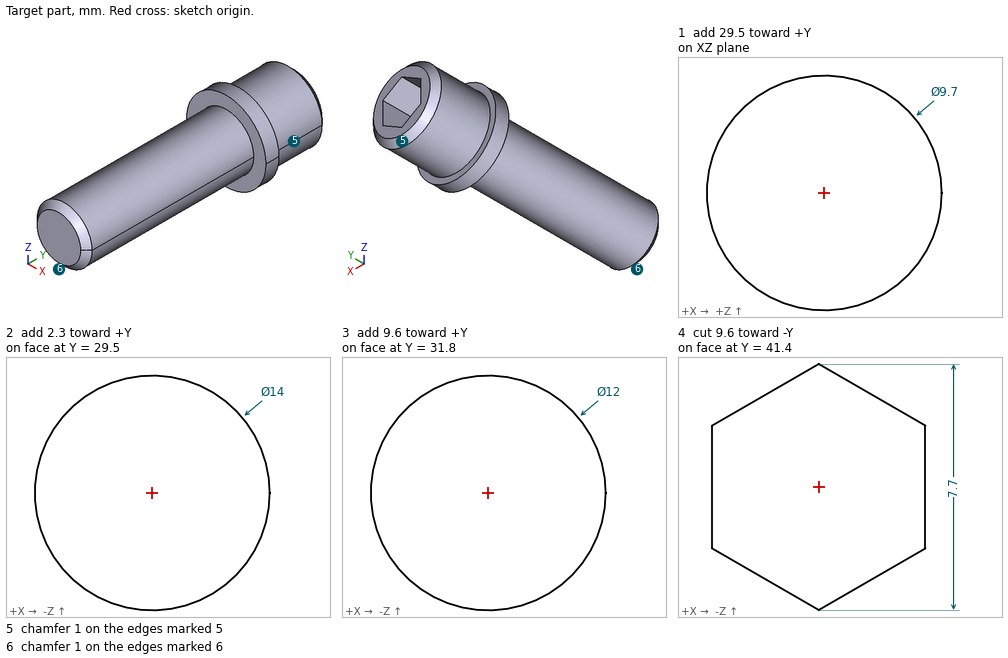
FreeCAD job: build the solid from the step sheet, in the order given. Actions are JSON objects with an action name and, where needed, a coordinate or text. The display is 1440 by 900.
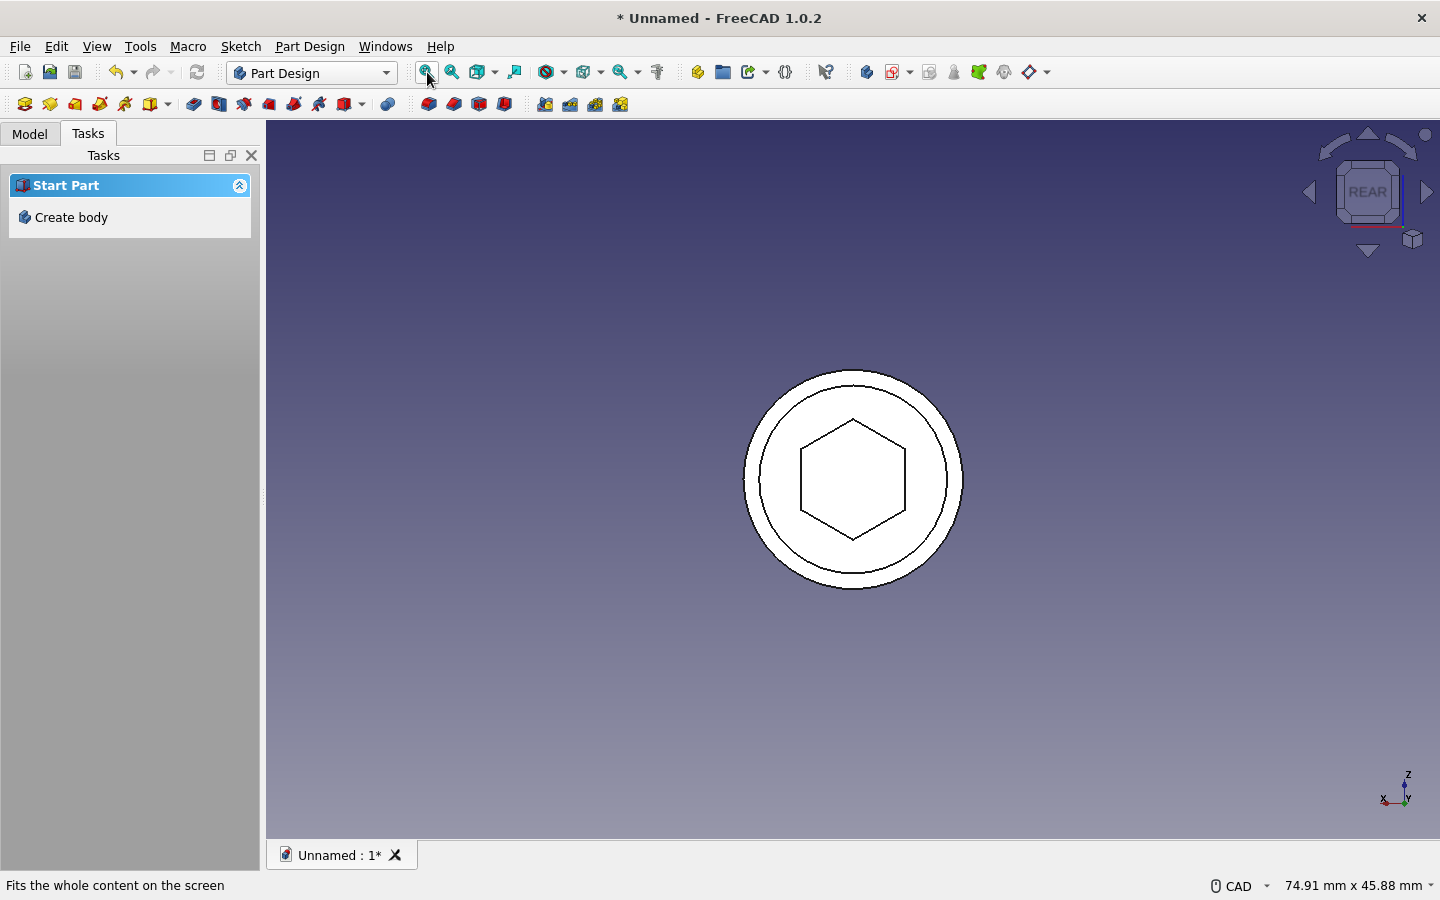
{"action": "left_click", "coordinate": [947, 478]}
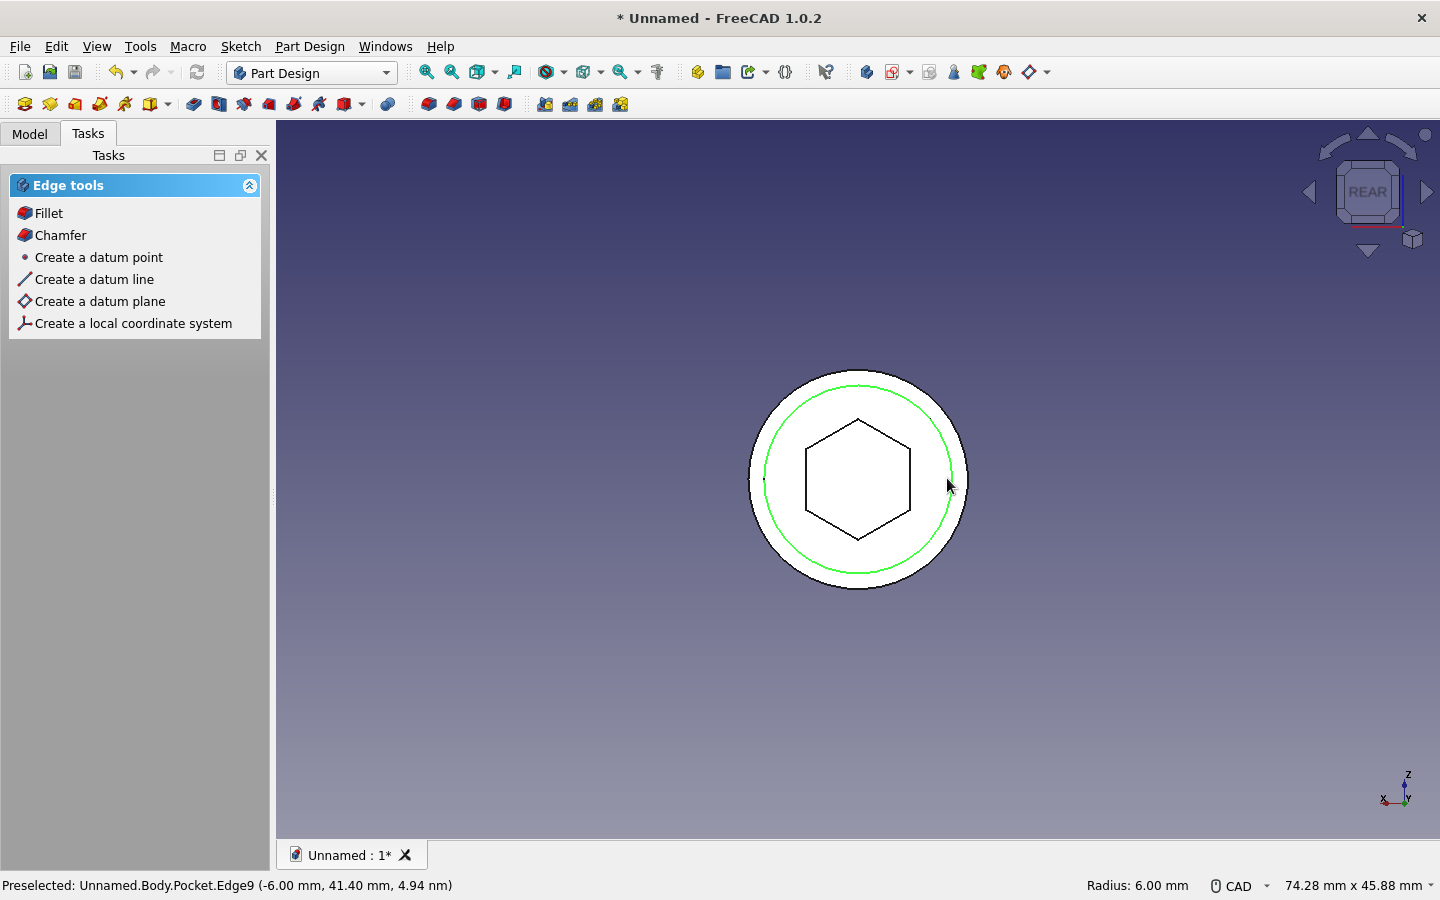
{"action": "left_click", "coordinate": [454, 104]}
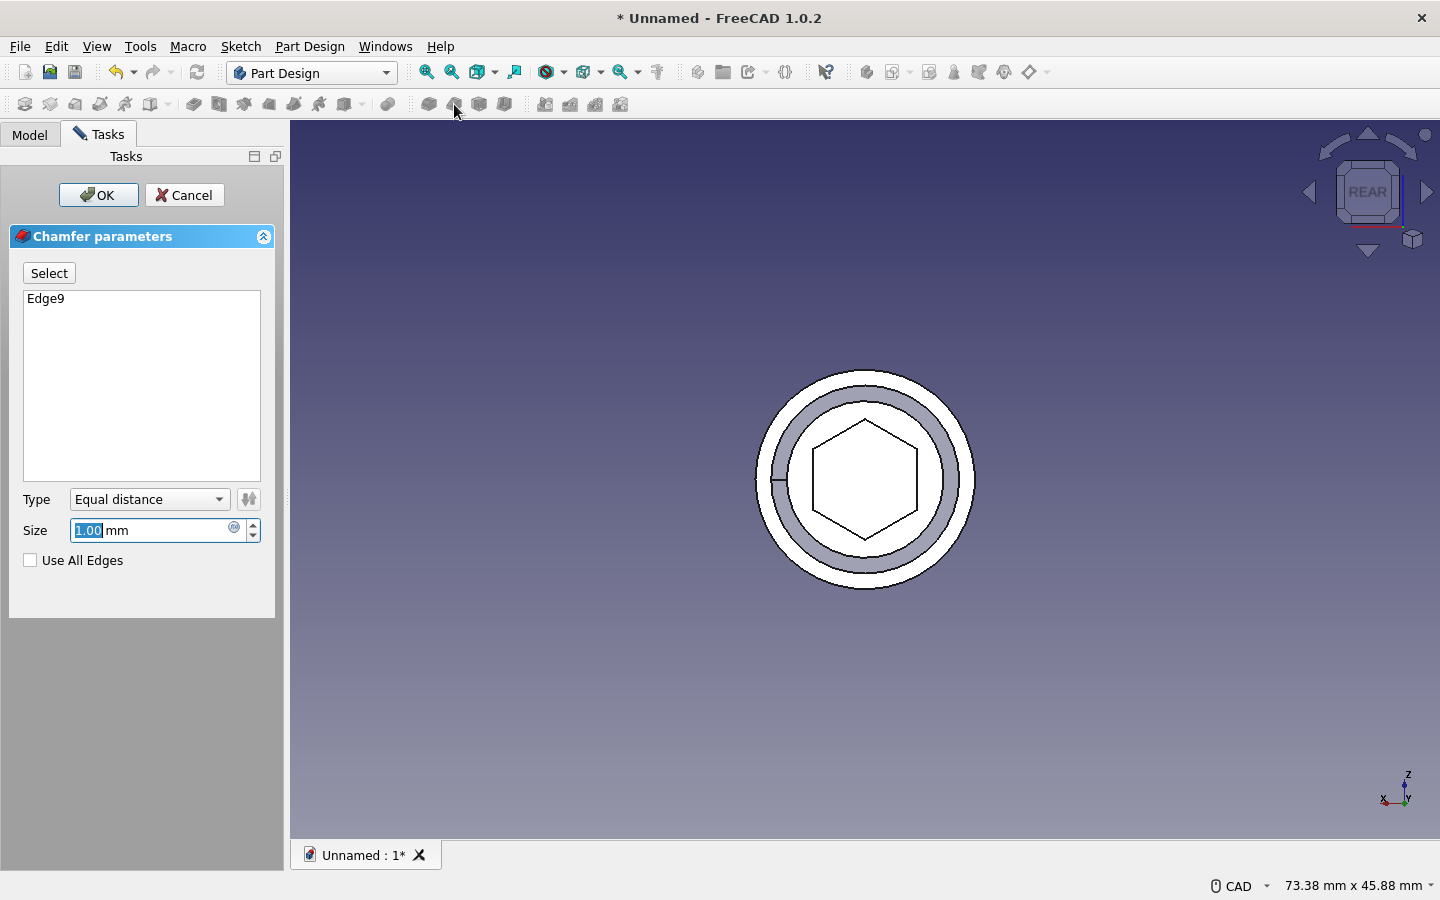
{"action": "type", "text": "1"}
{"action": "key", "text": "Tab"}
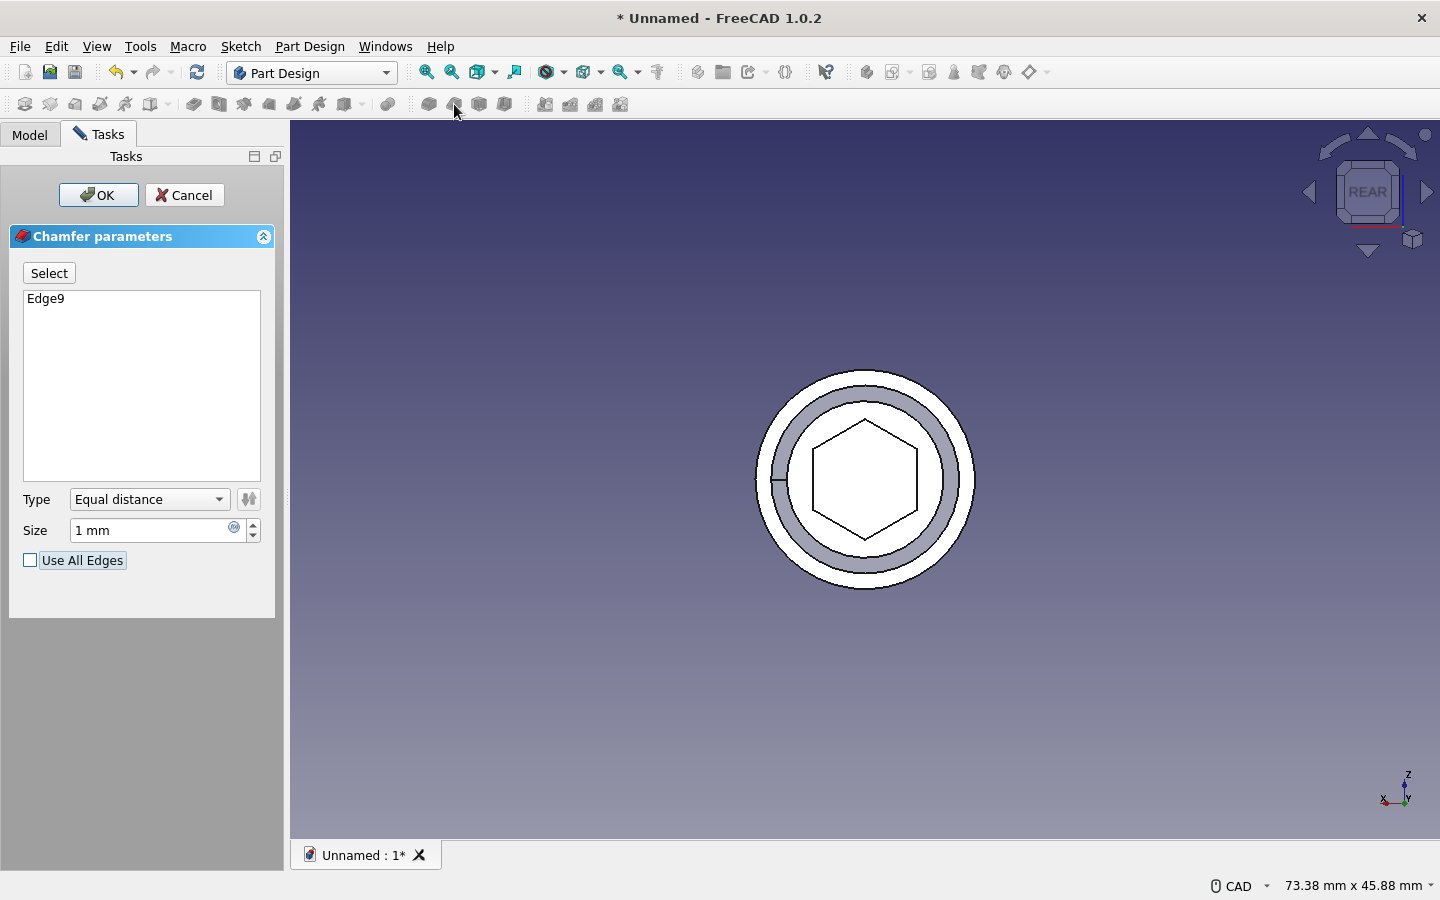
{"action": "left_click", "coordinate": [99, 195]}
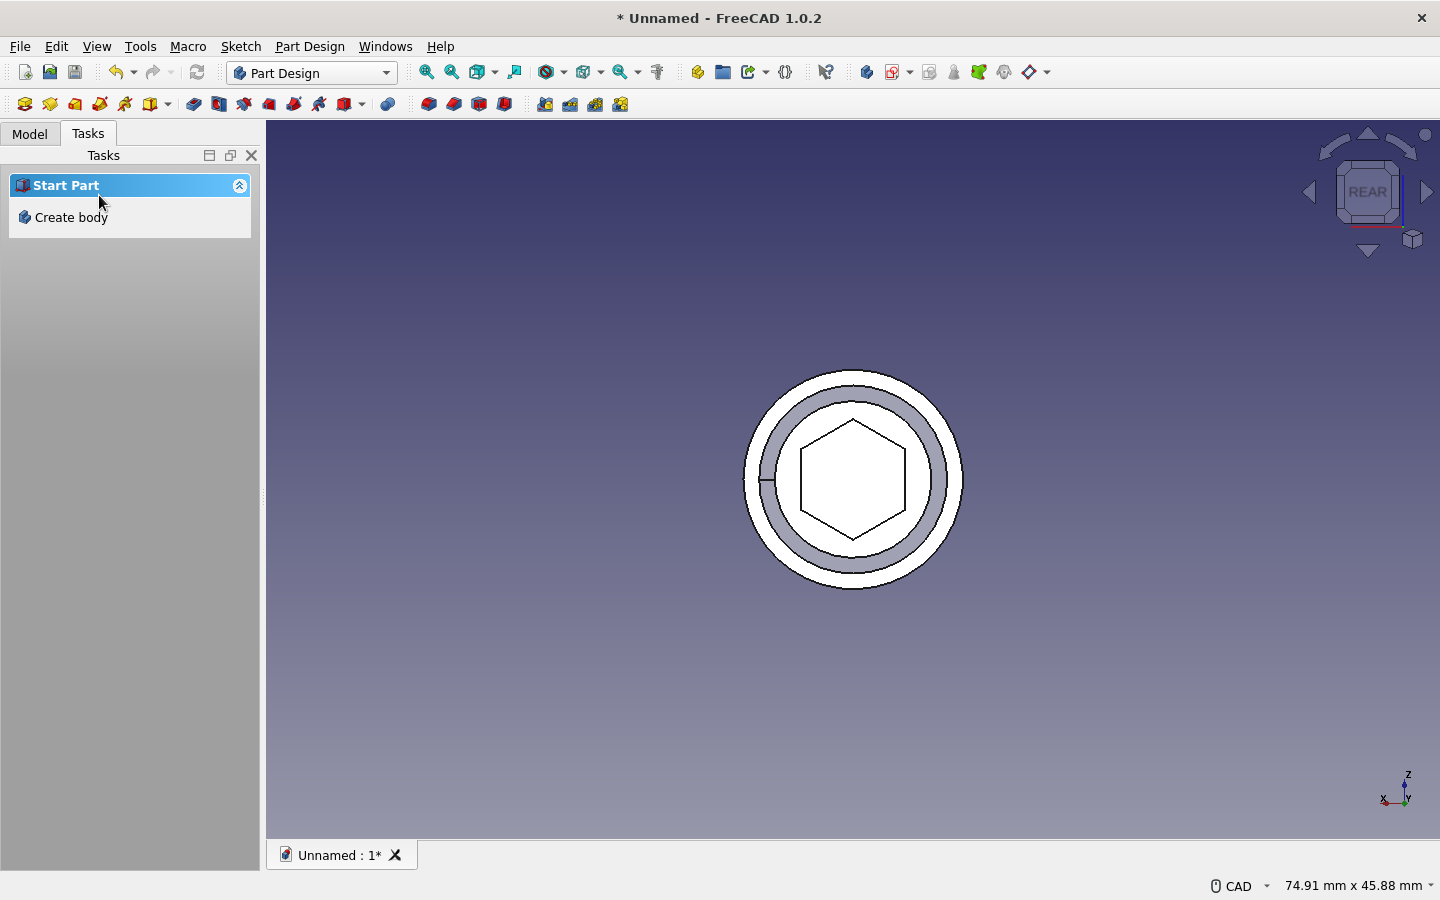
{"action": "left_click", "coordinate": [427, 72]}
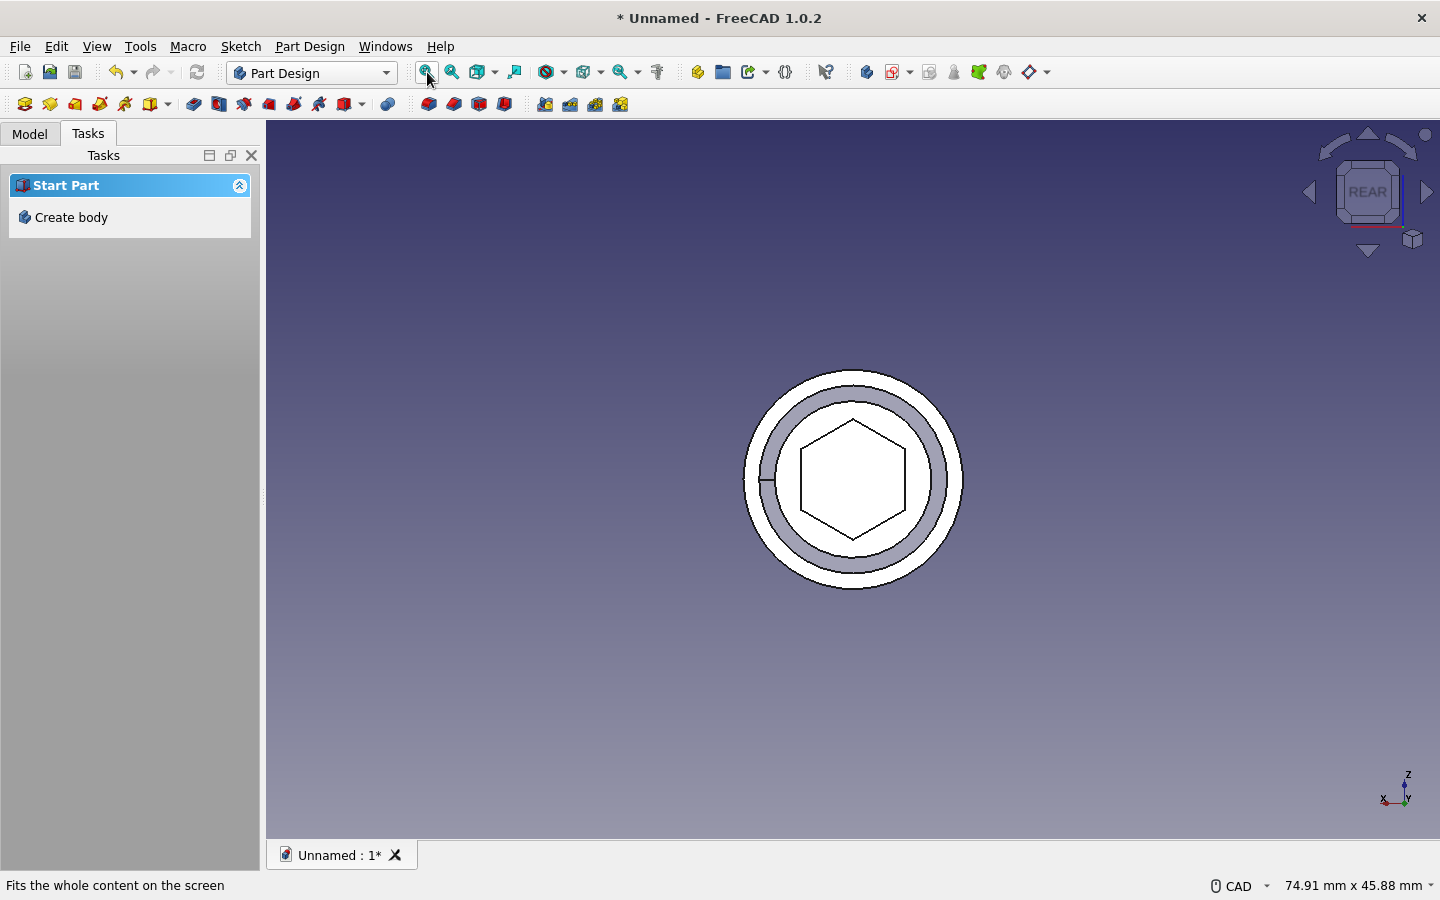
{"action": "key", "text": "0"}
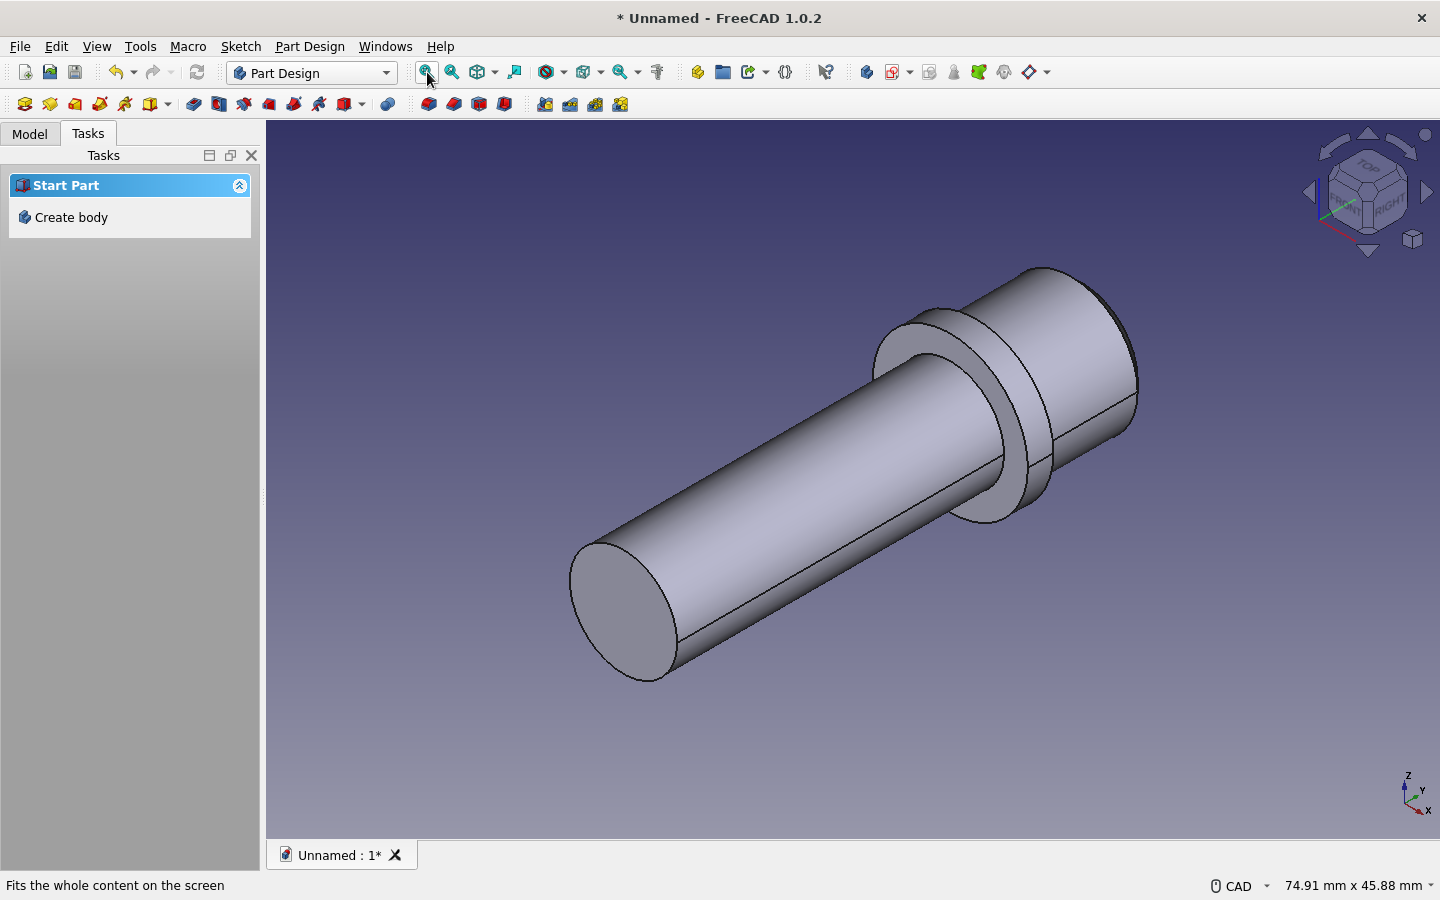
{"action": "left_click", "coordinate": [580, 549]}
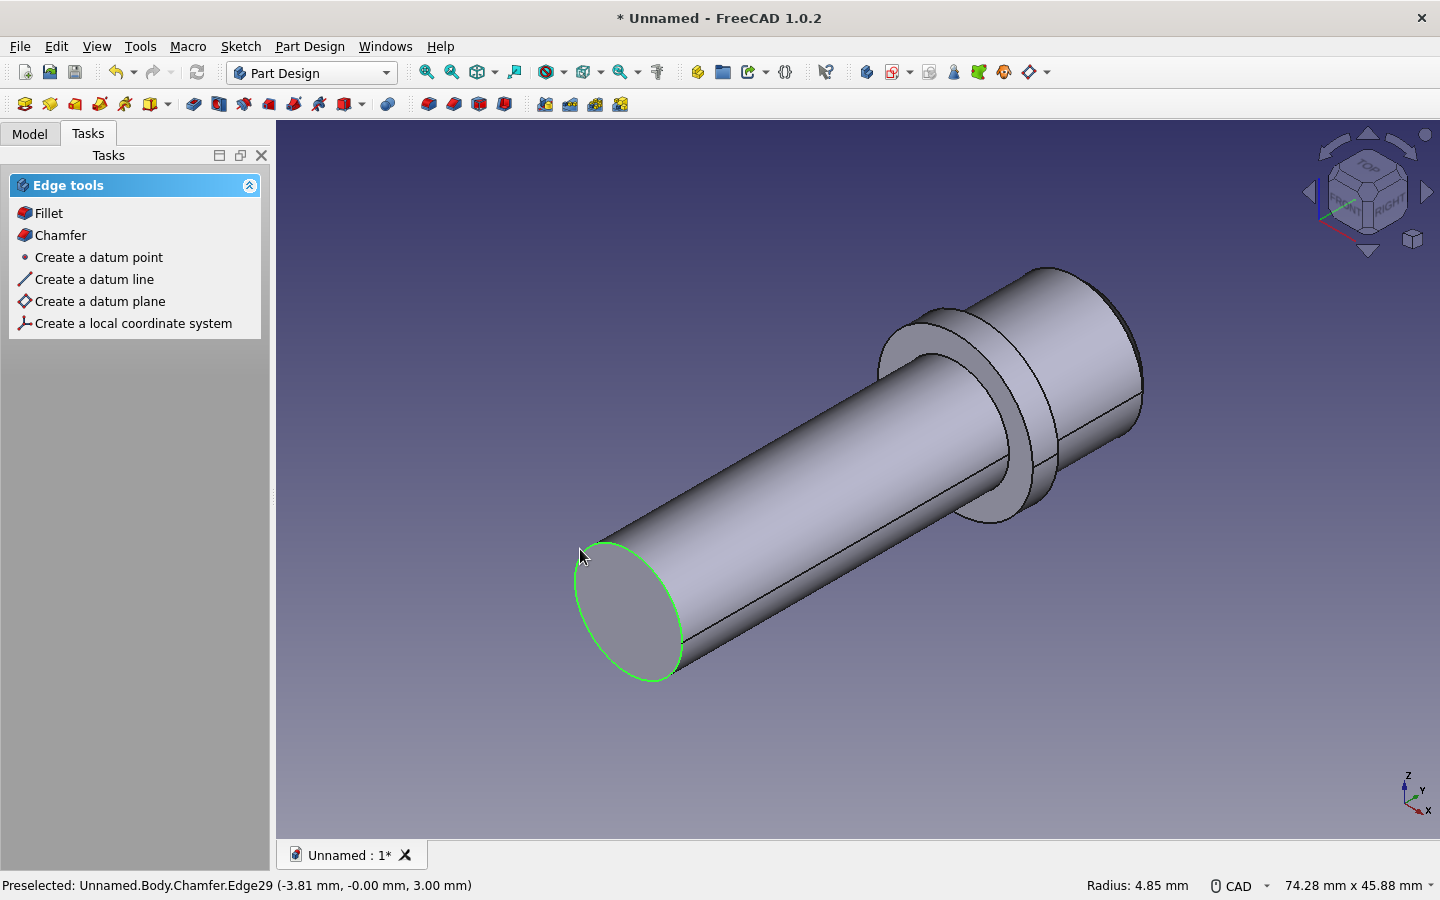
{"action": "left_click", "coordinate": [454, 104]}